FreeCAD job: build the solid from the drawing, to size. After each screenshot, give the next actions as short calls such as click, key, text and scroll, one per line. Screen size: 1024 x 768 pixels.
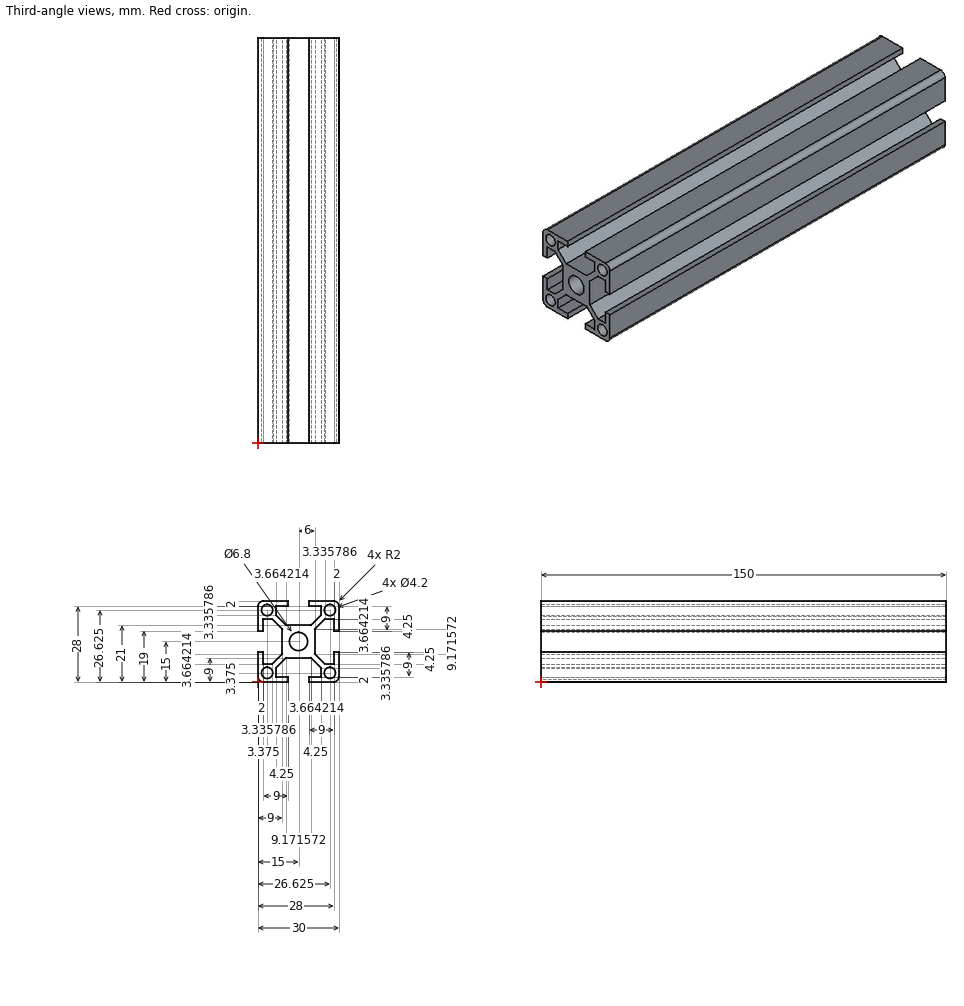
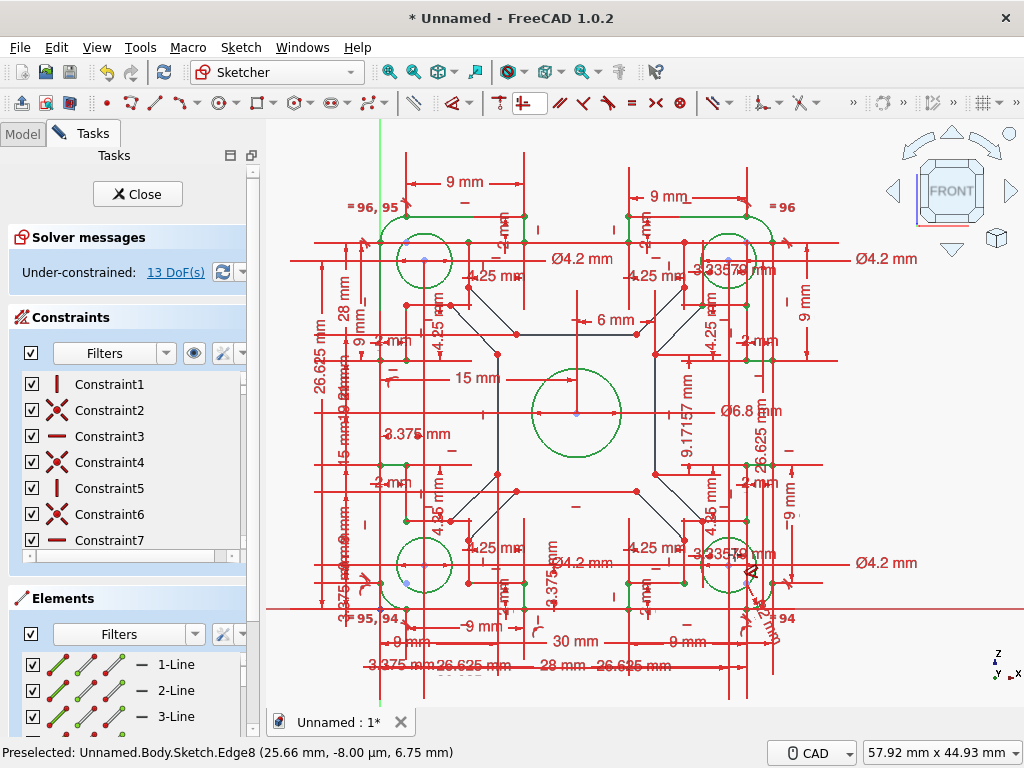
click(684, 570)
click(790, 577)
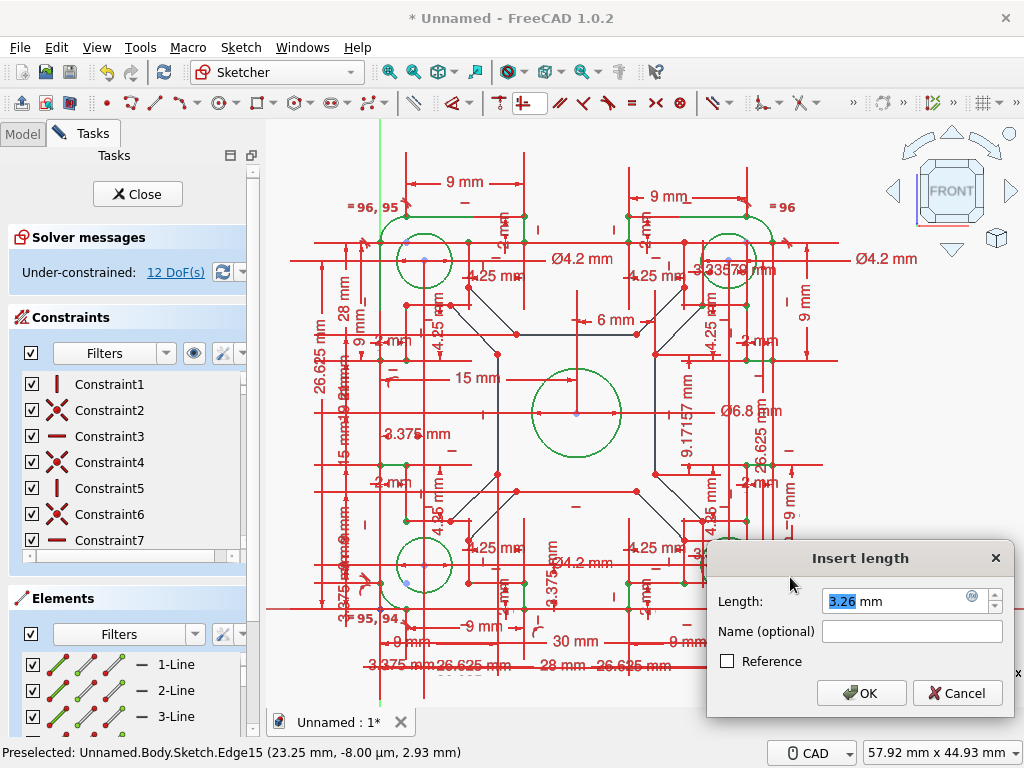
text(3.335786)
key(Return)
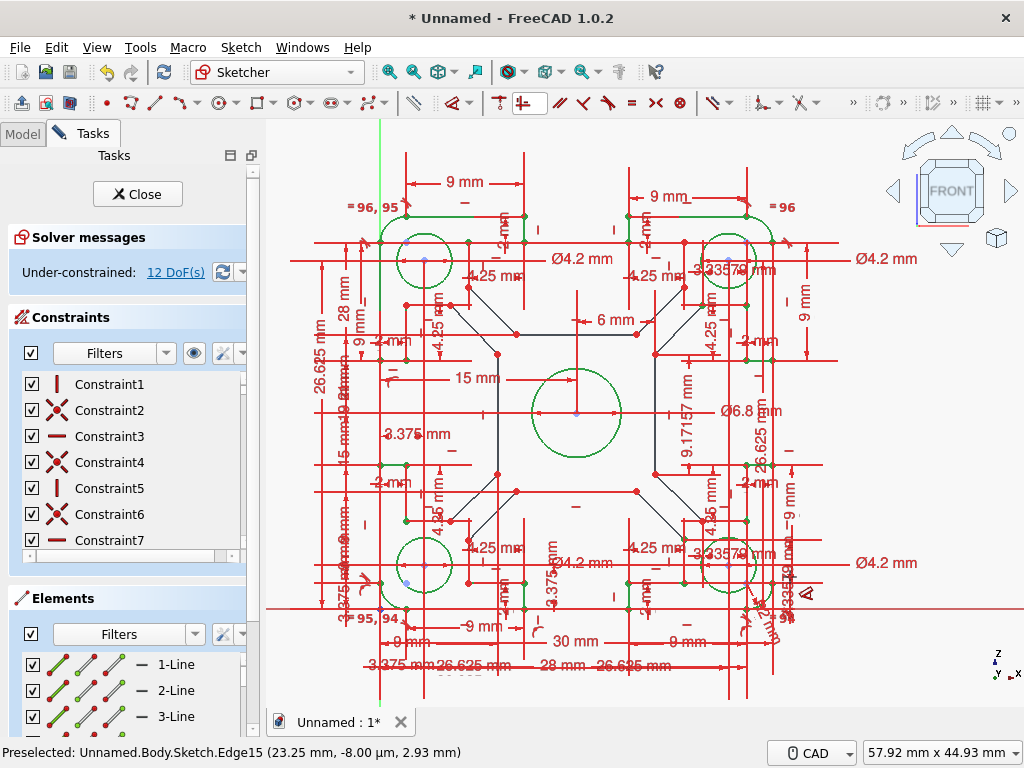
click(600, 492)
click(576, 526)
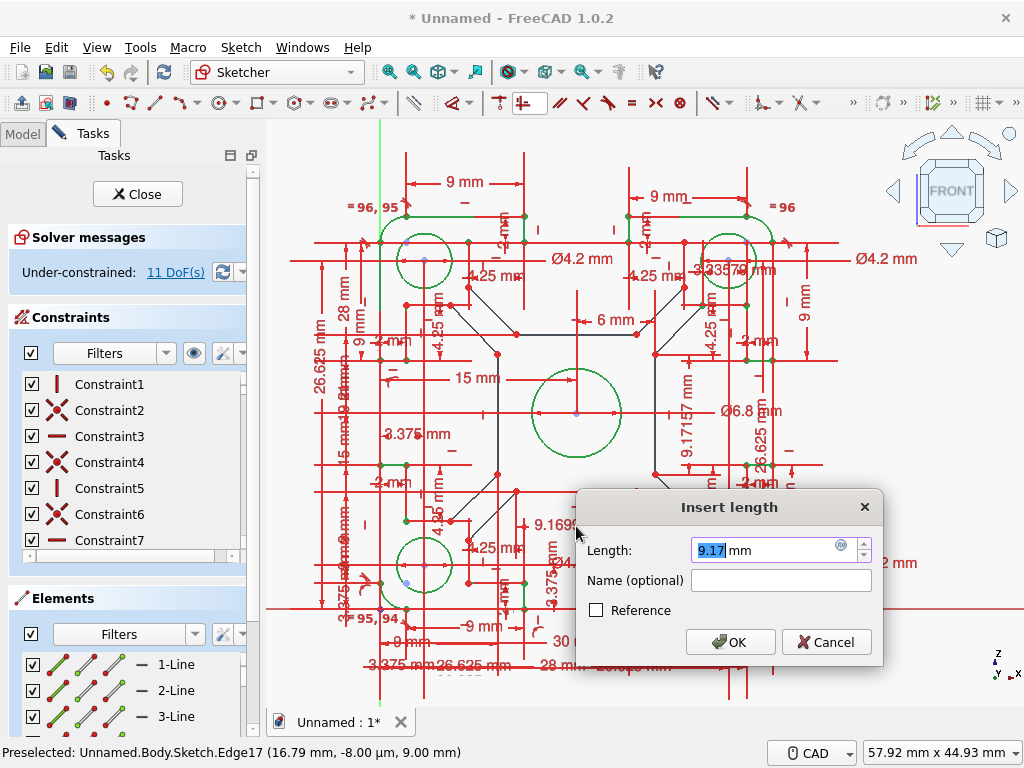
text(9.171572)
key(Return)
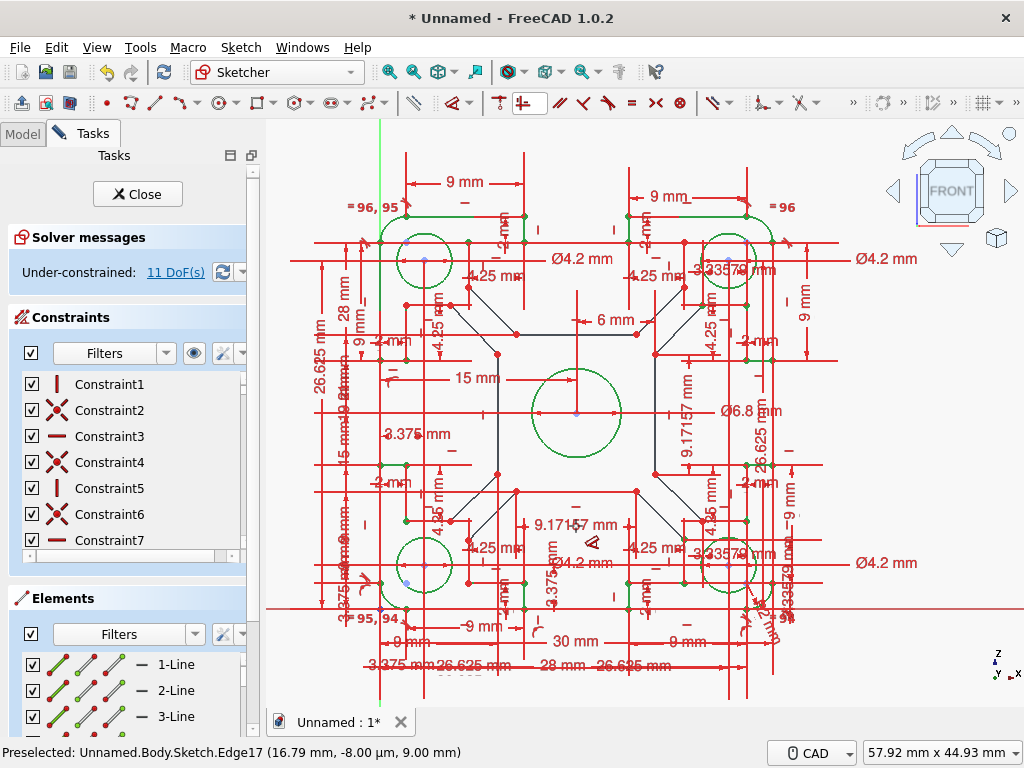
click(469, 553)
click(435, 572)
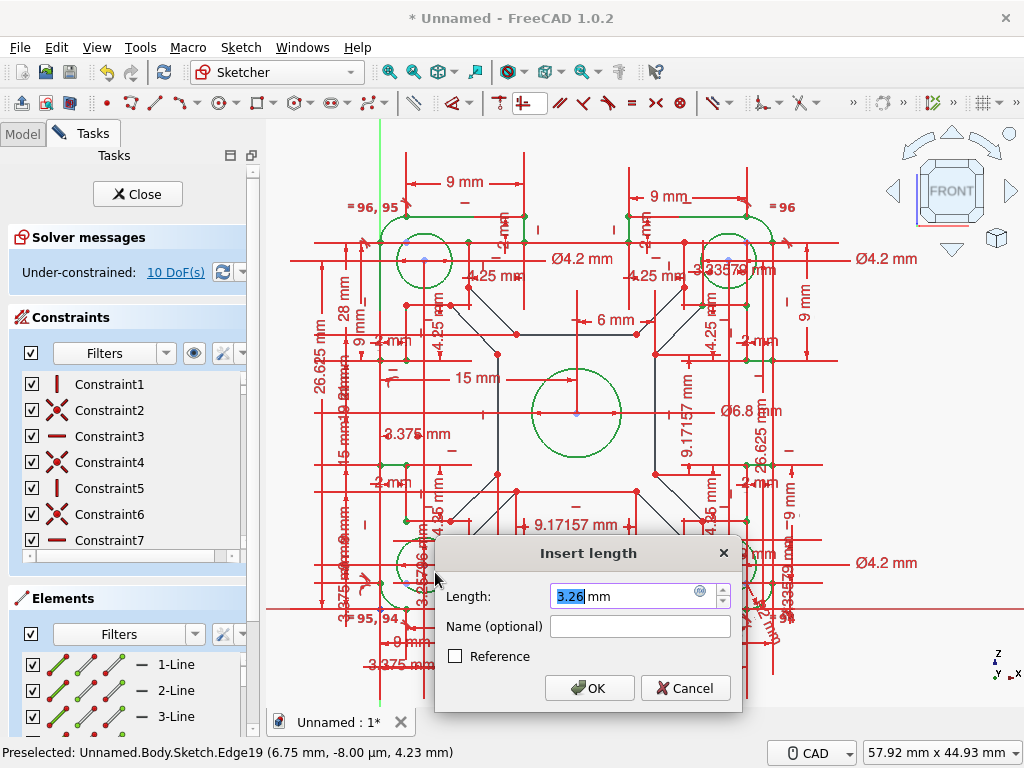
text(3.335786)
key(Return)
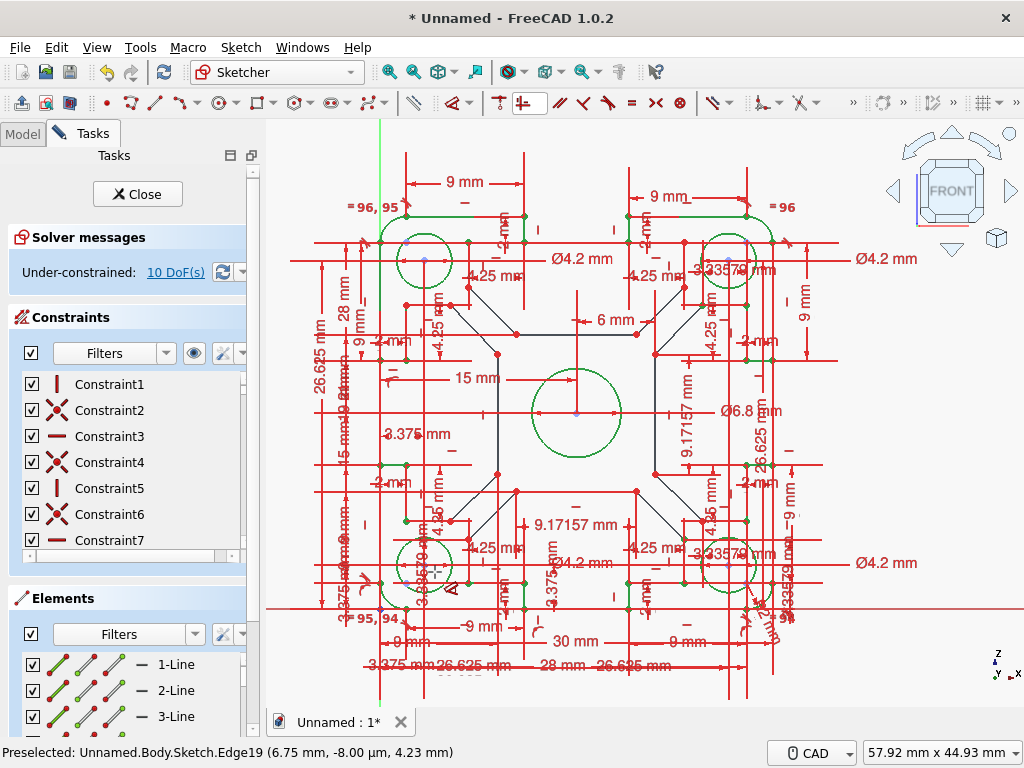
click(420, 521)
click(428, 463)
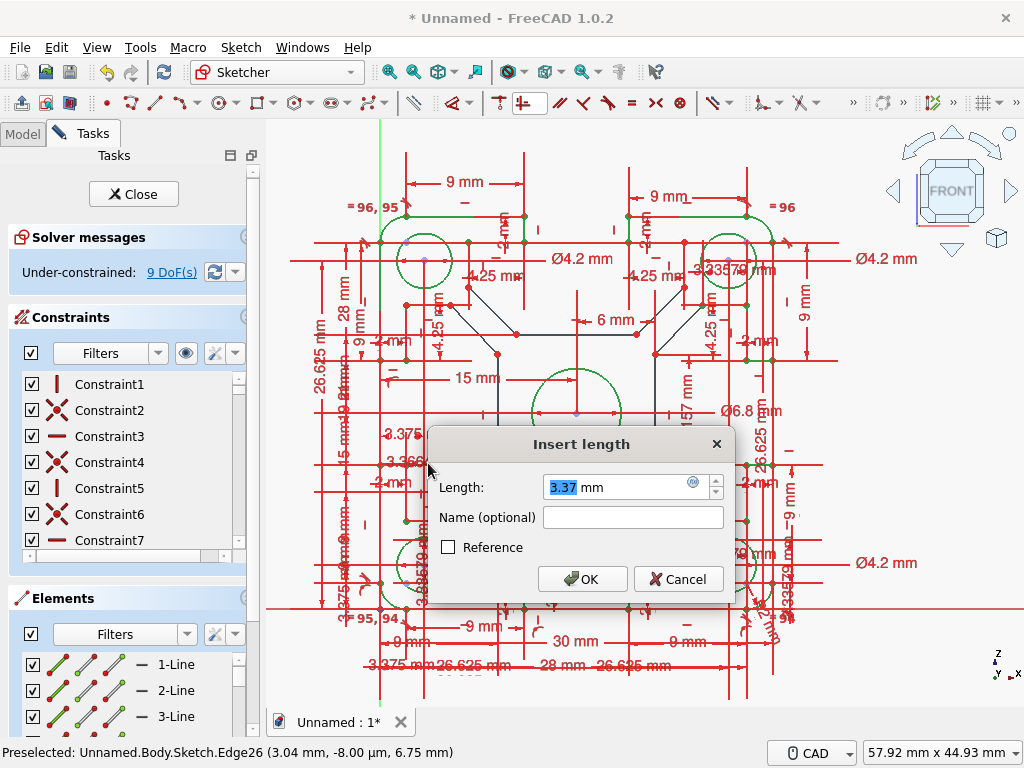
text(3.335786)
key(Return)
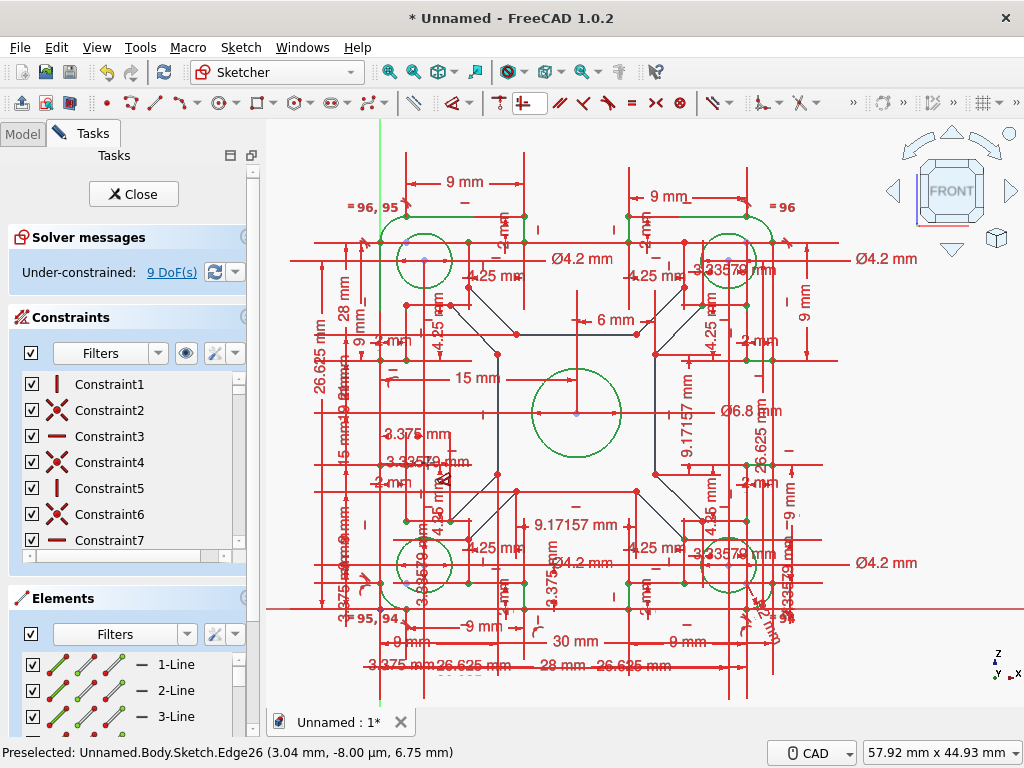
click(498, 439)
click(464, 415)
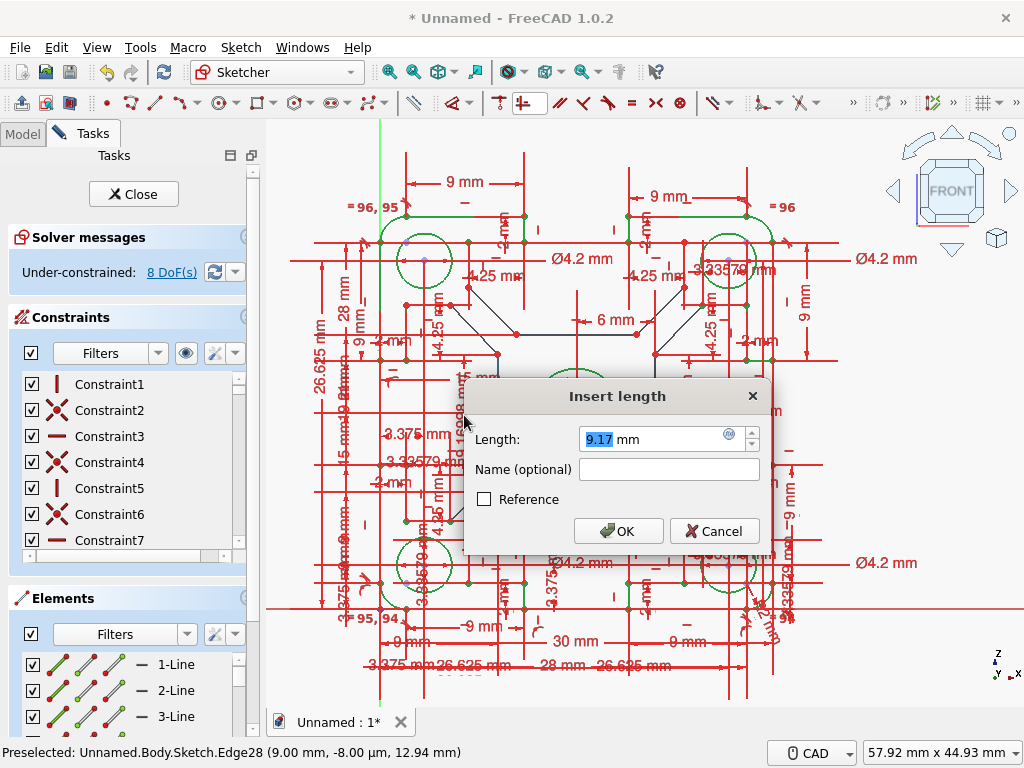
text(9.171572)
key(Return)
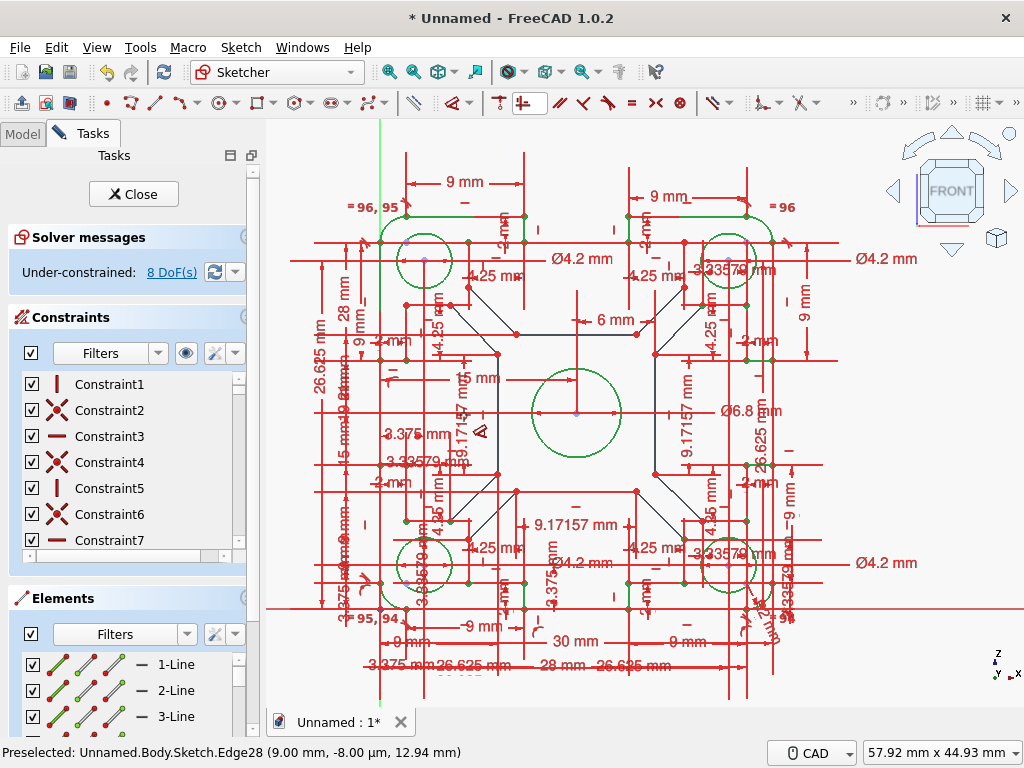
click(437, 305)
click(418, 271)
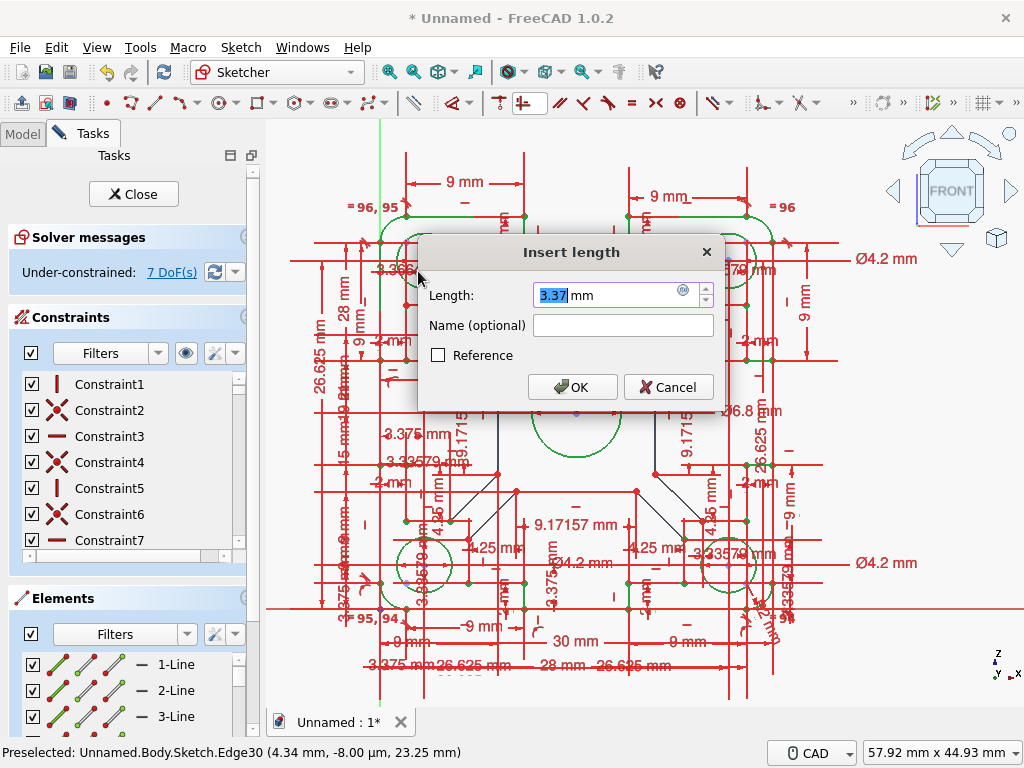
text(3.335786)
key(Return)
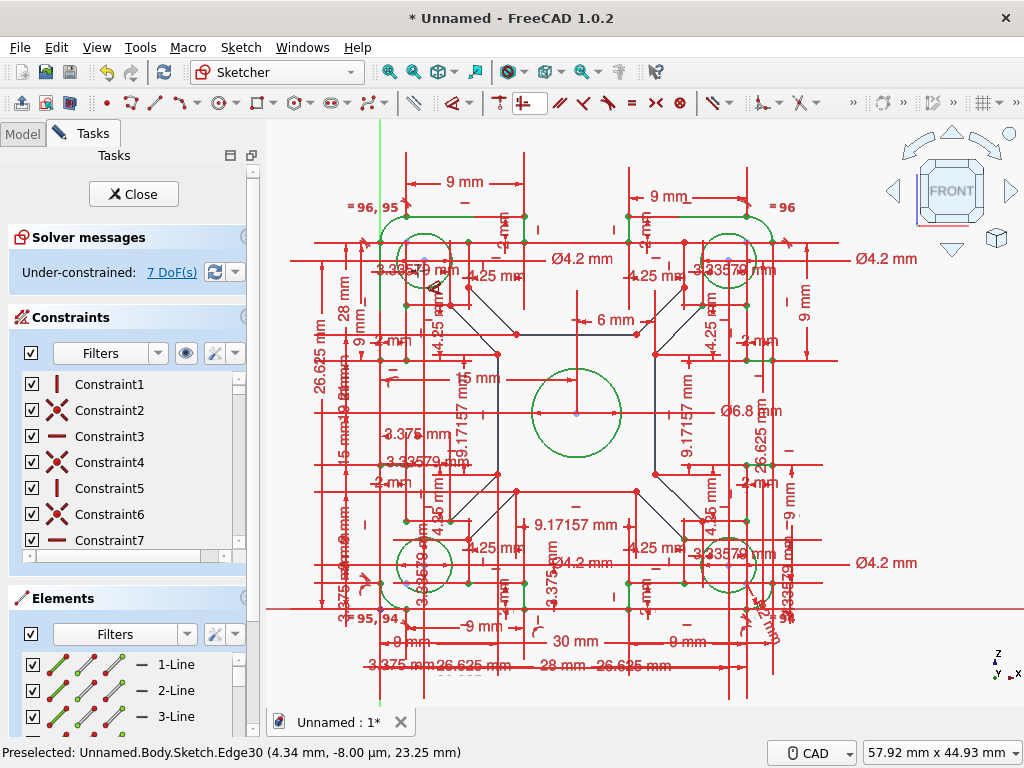
click(469, 256)
click(551, 255)